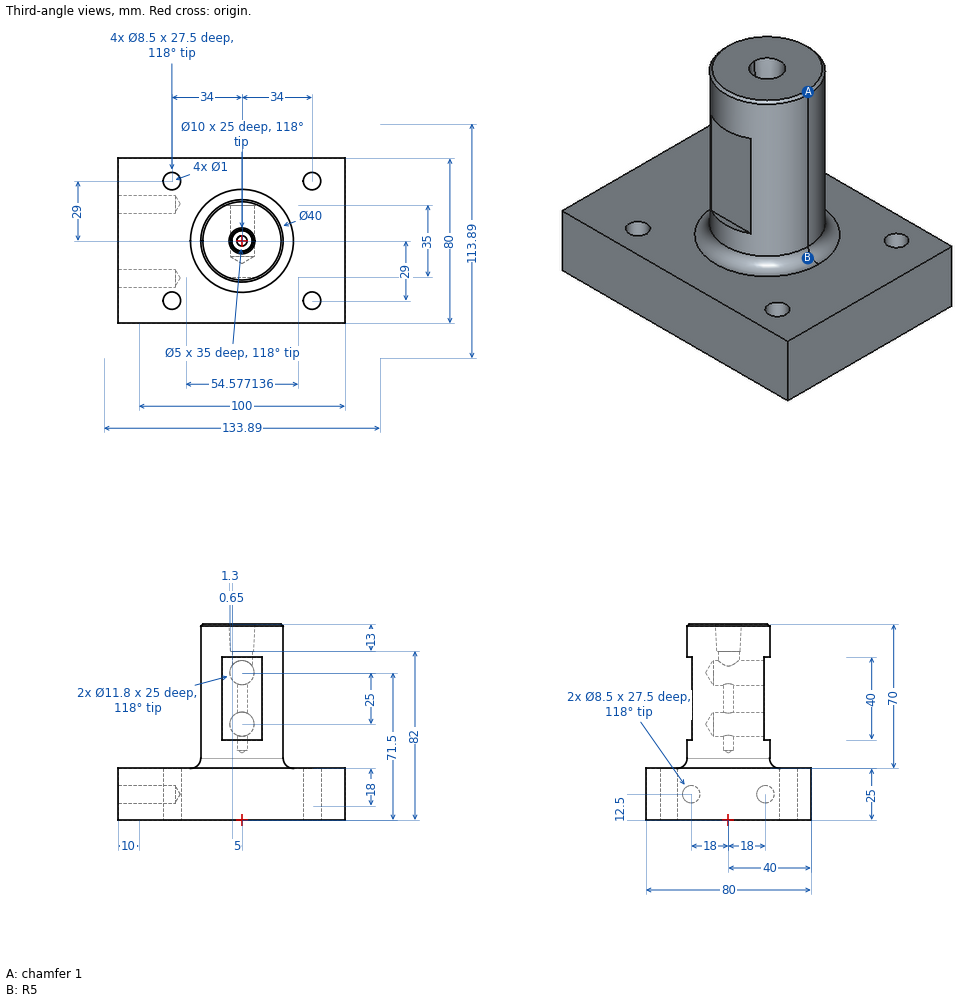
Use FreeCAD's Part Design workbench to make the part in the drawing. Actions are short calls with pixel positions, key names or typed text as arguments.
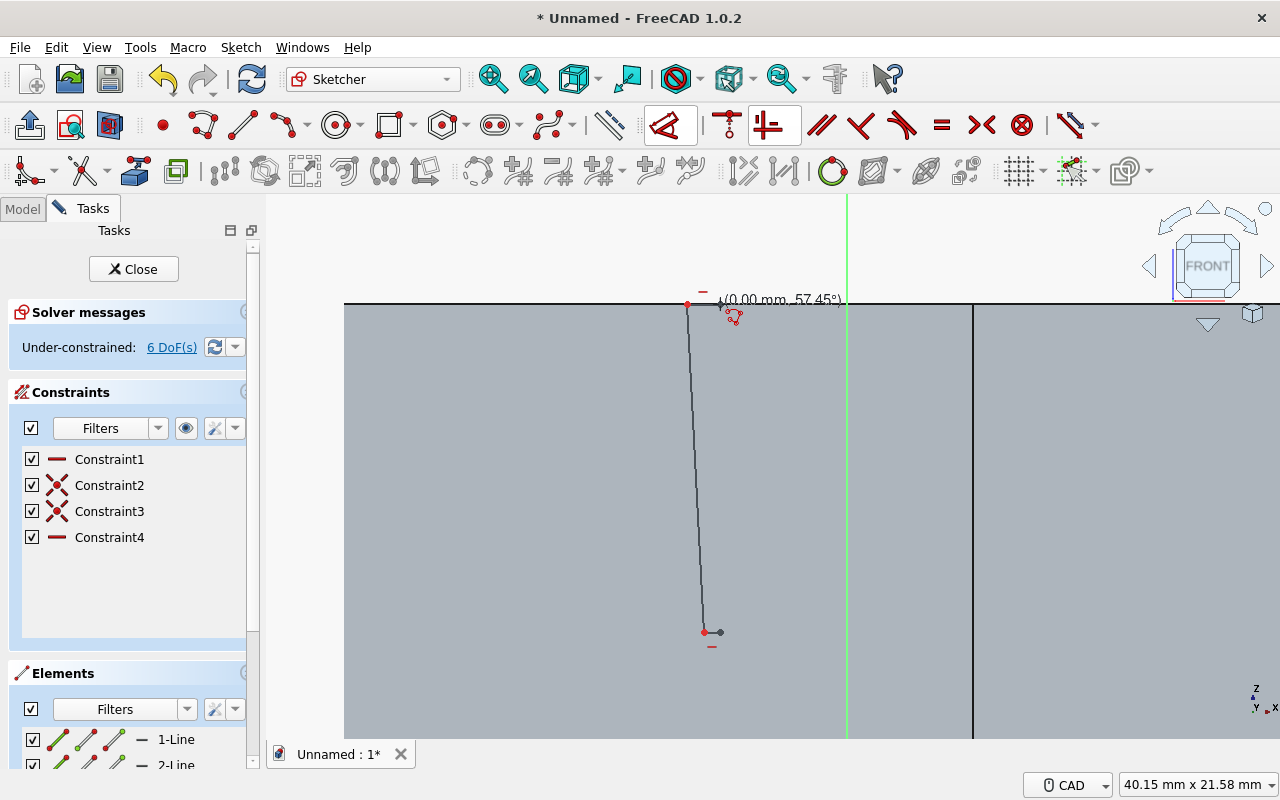
scroll(720, 632, up, 4)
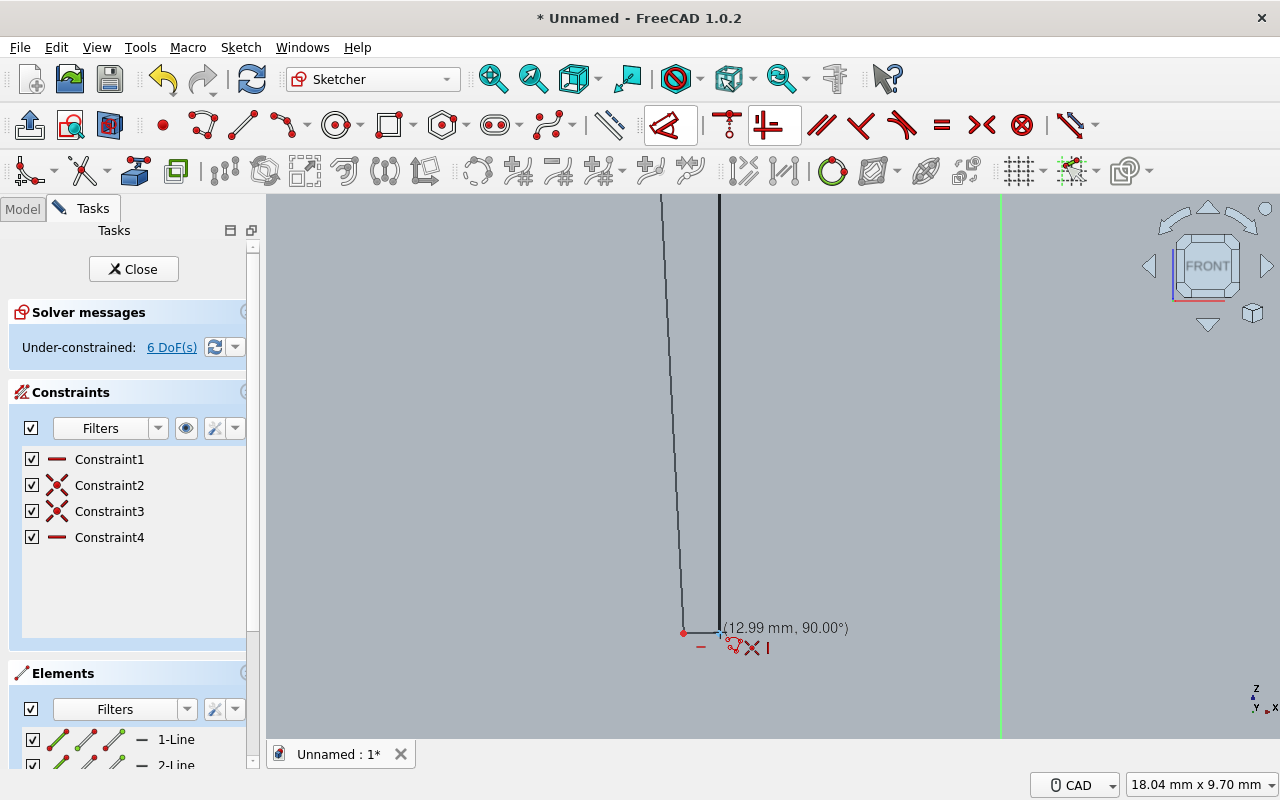
click(719, 633)
key(Escape)
key(Escape)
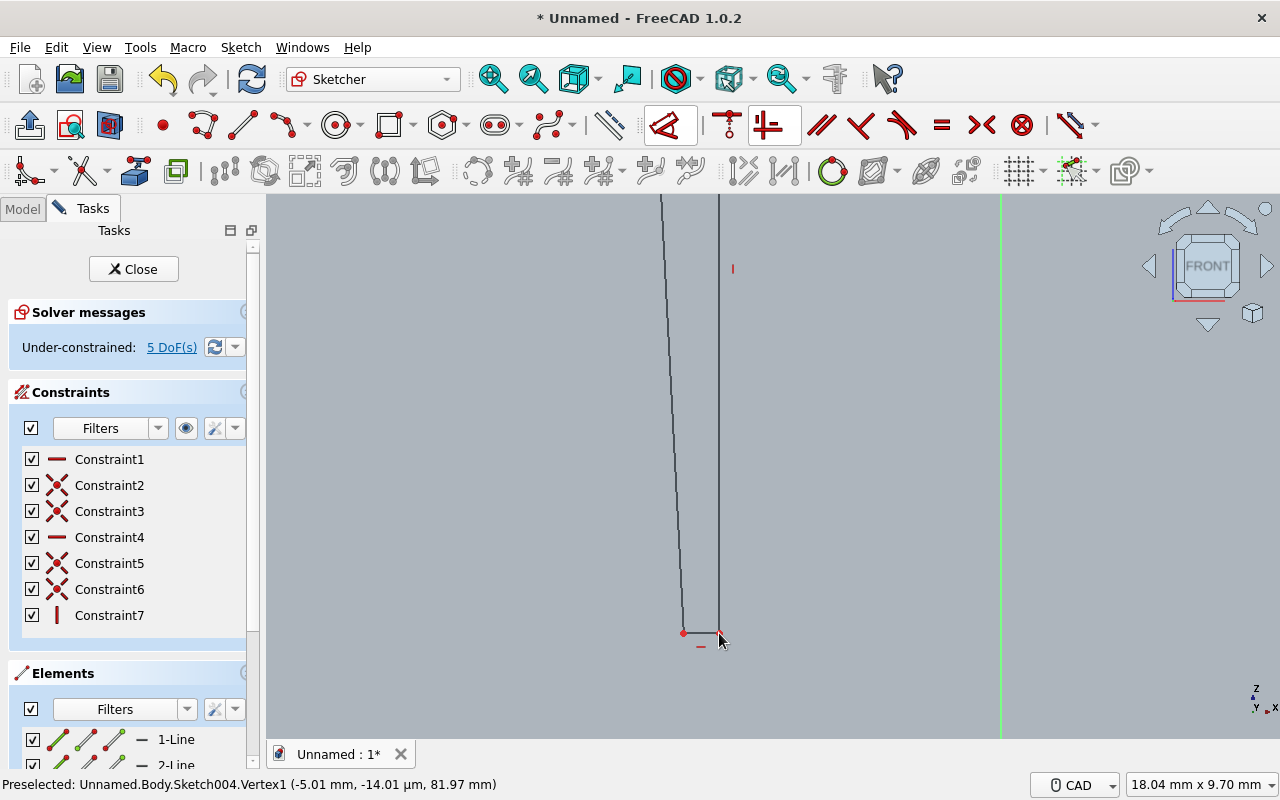
click(719, 414)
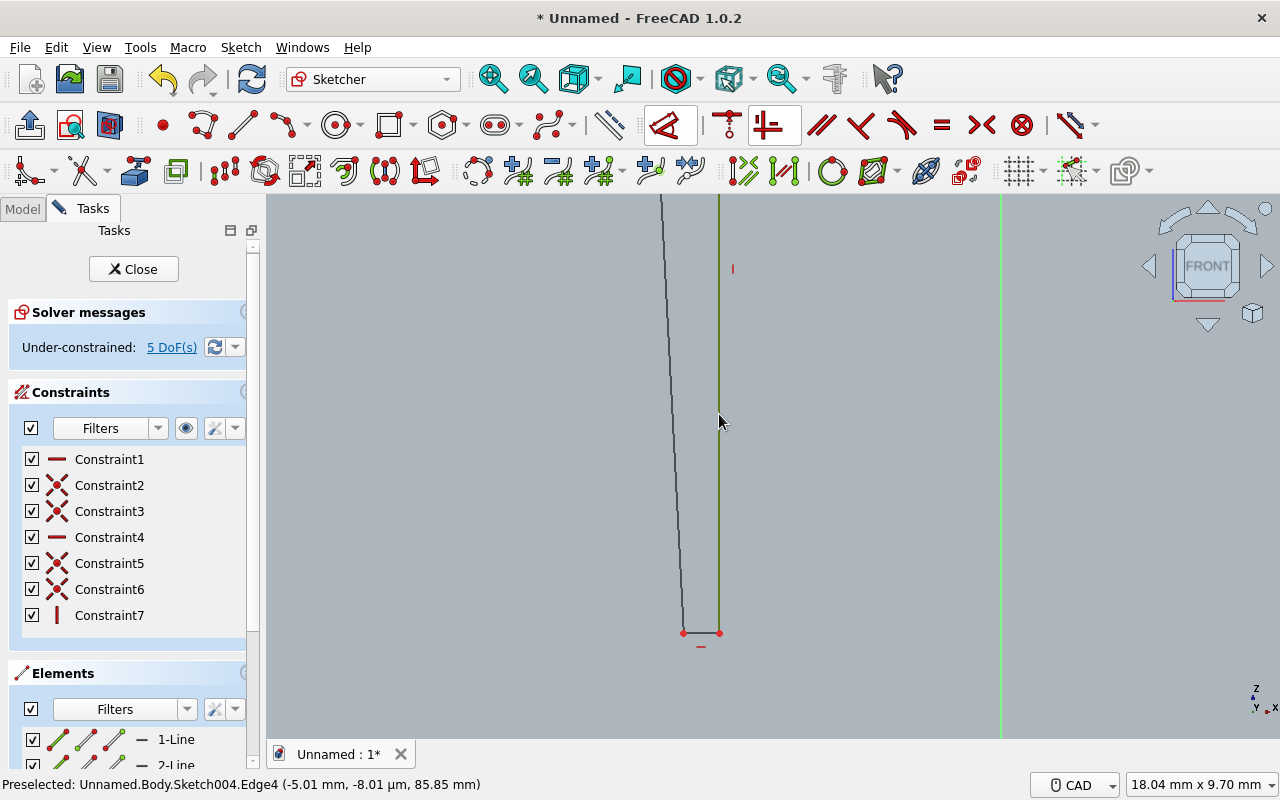
click(692, 126)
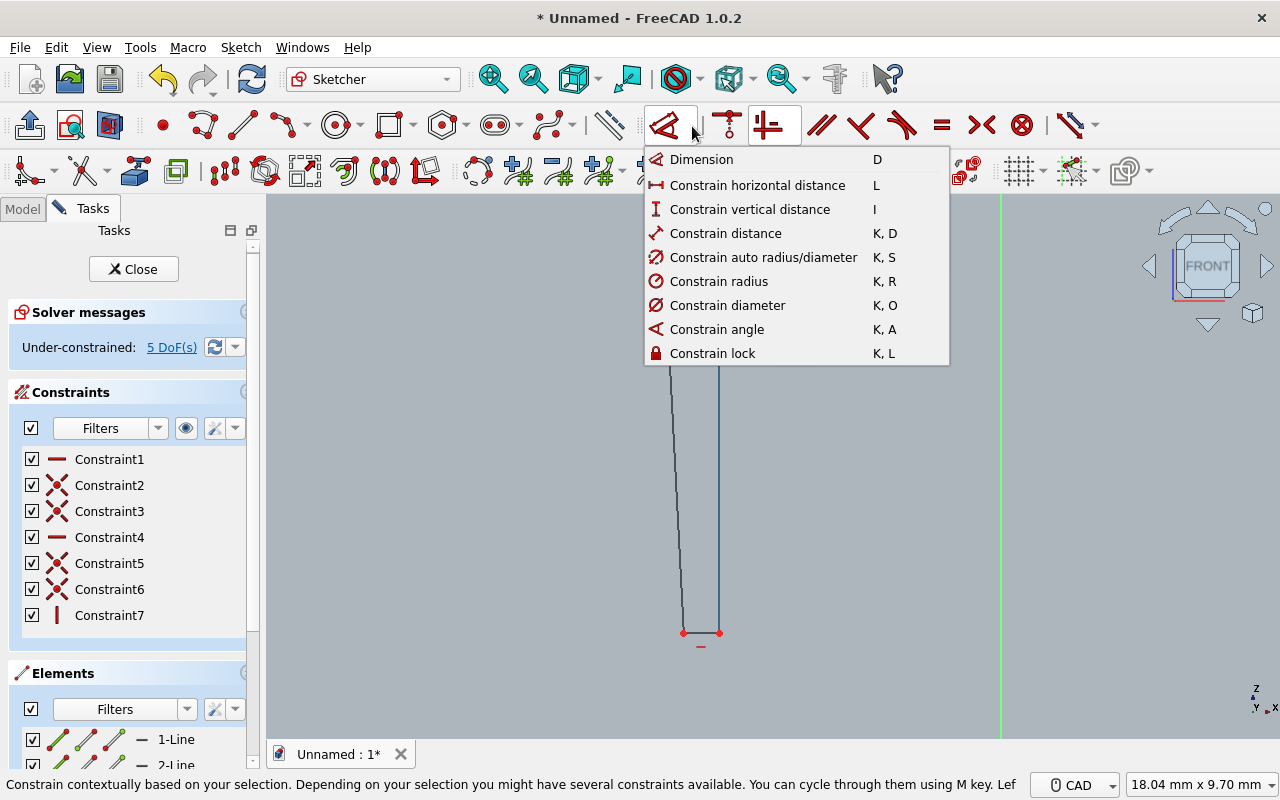
click(797, 209)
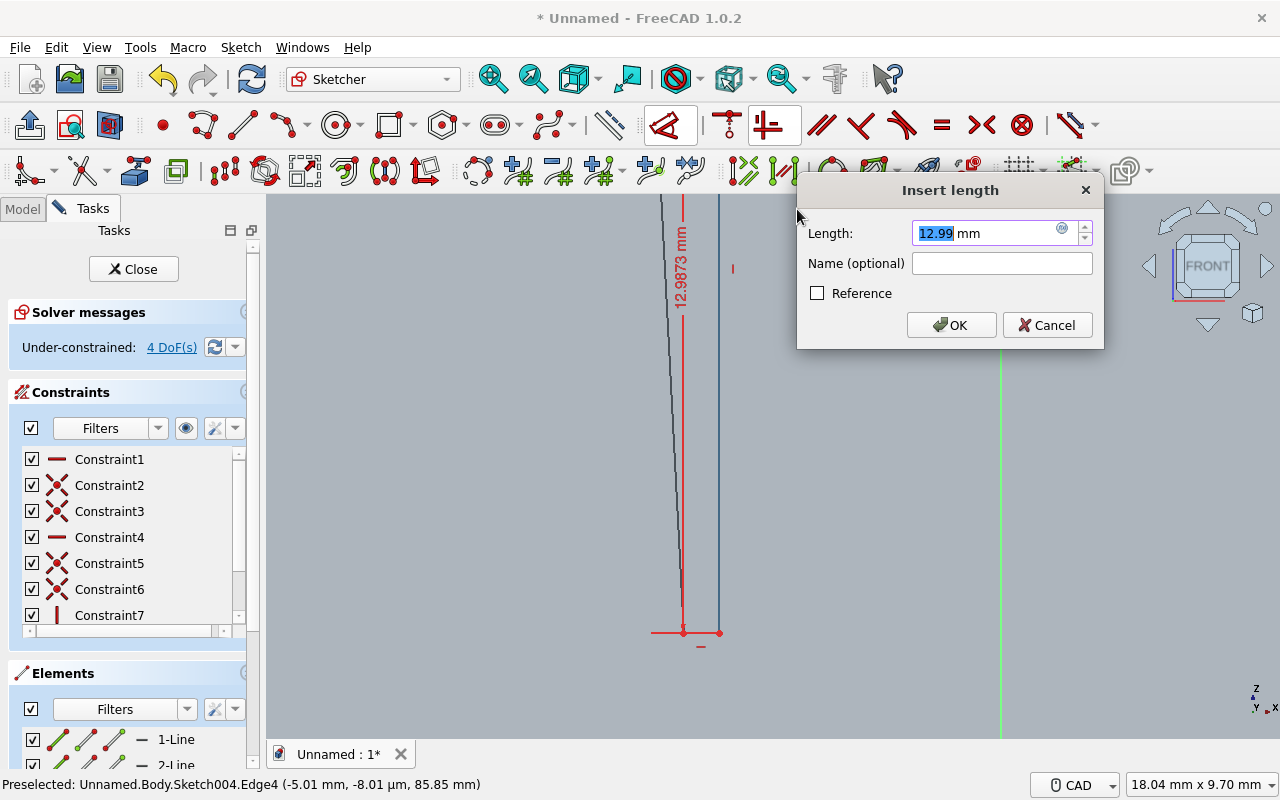
text(13)
key(Return)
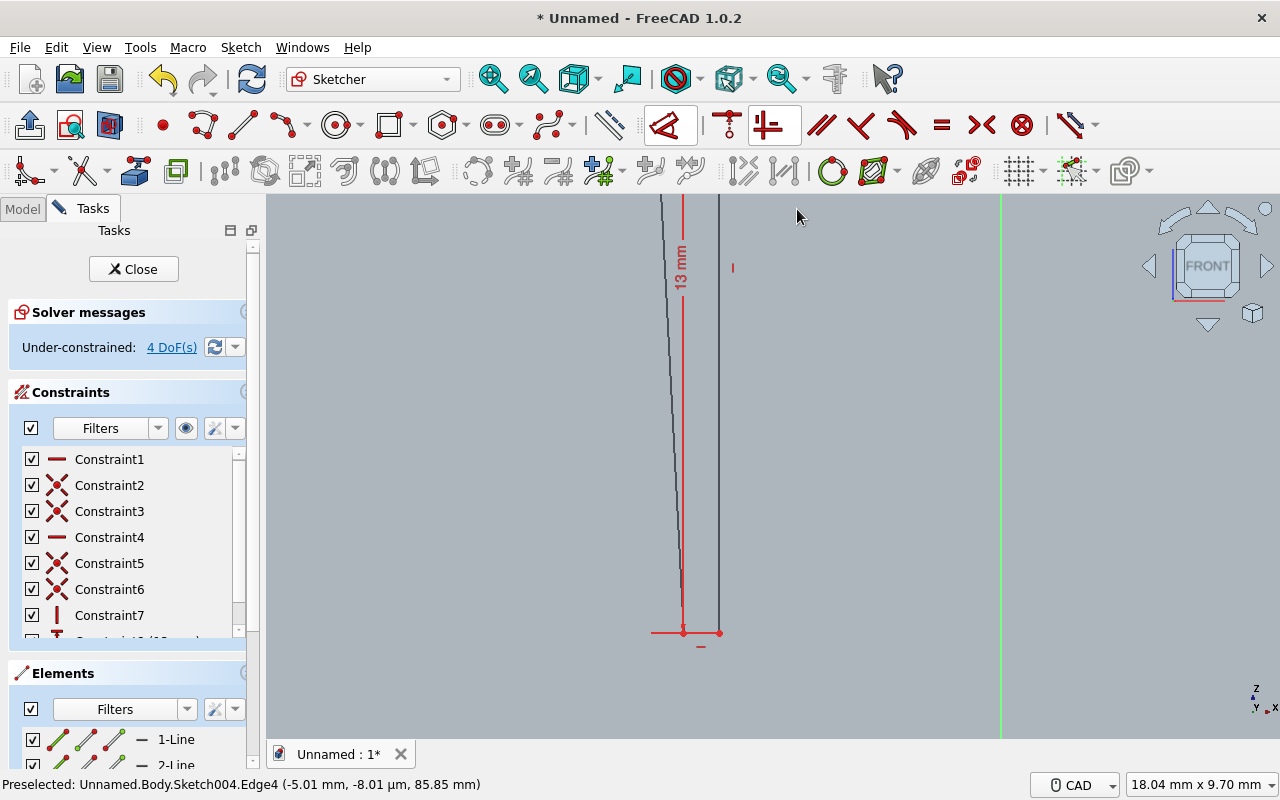
click(719, 633)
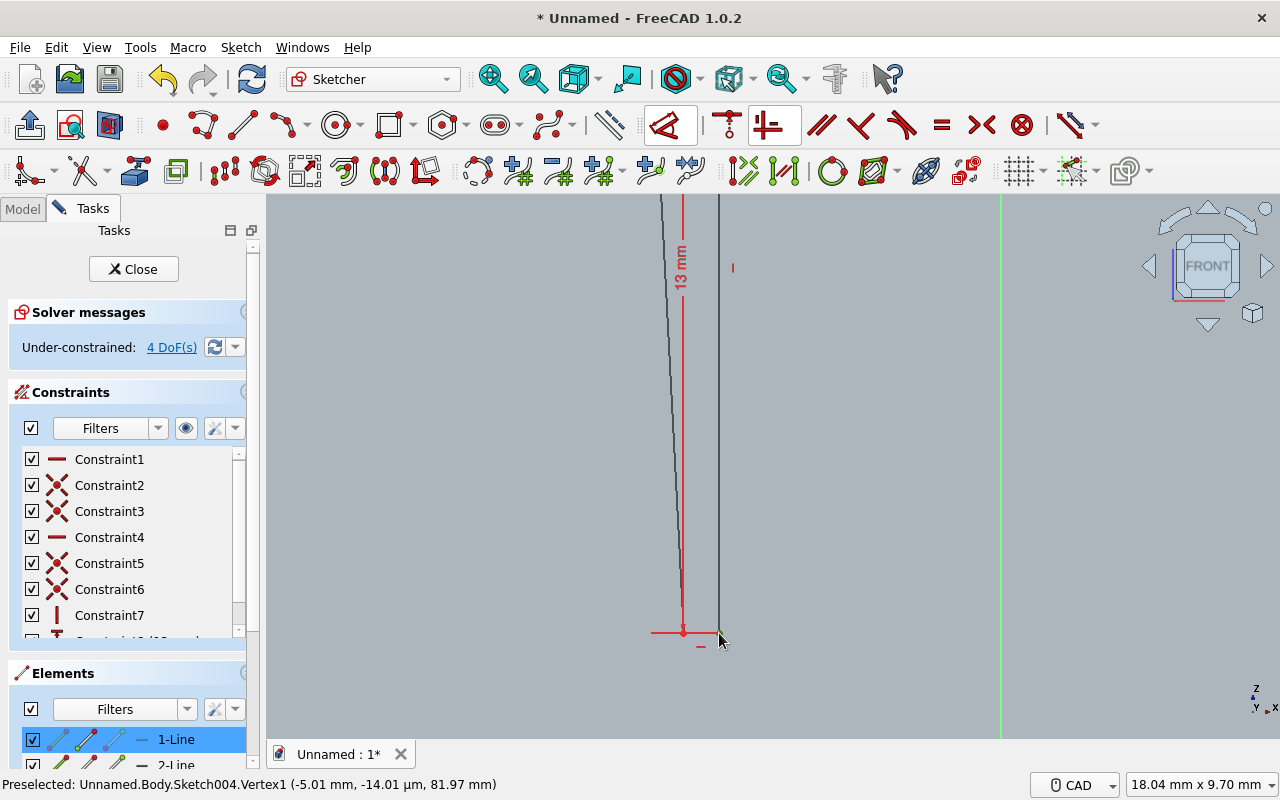
click(692, 126)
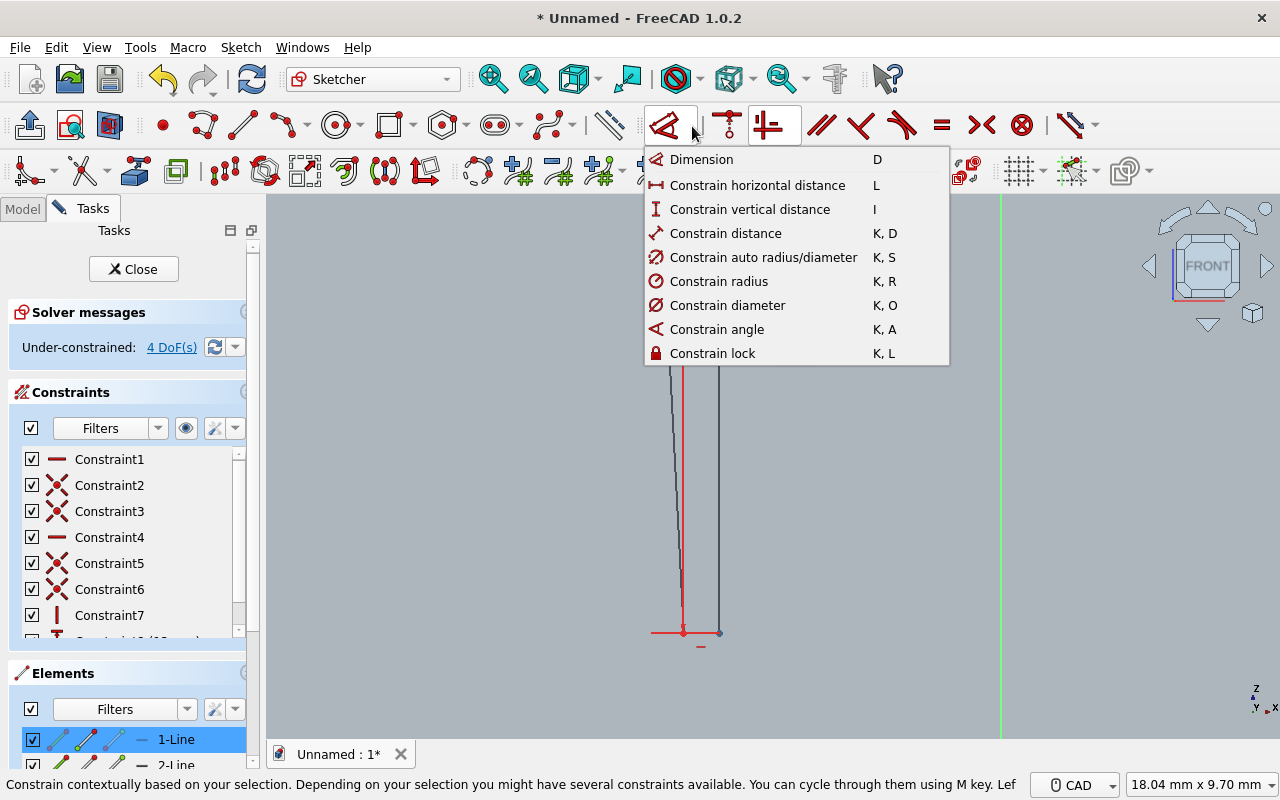
click(797, 185)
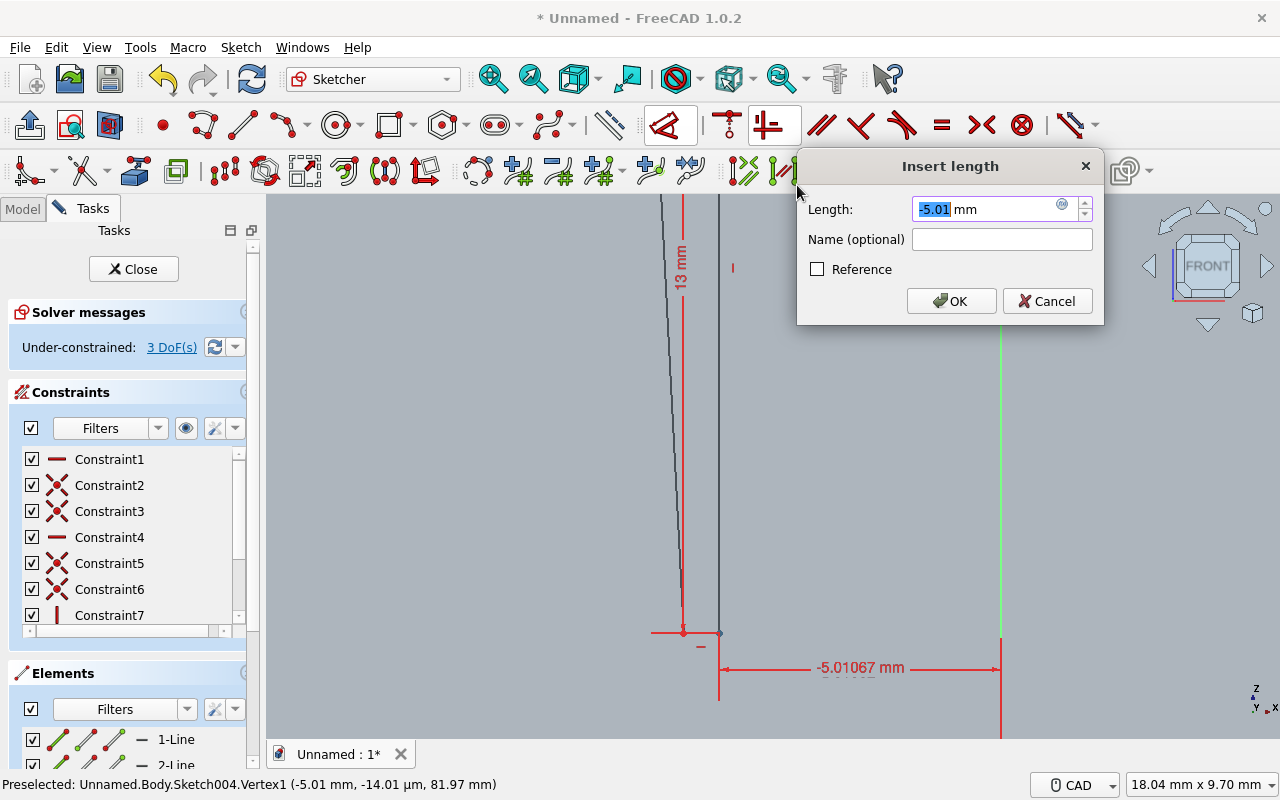
text(-5)
key(Return)